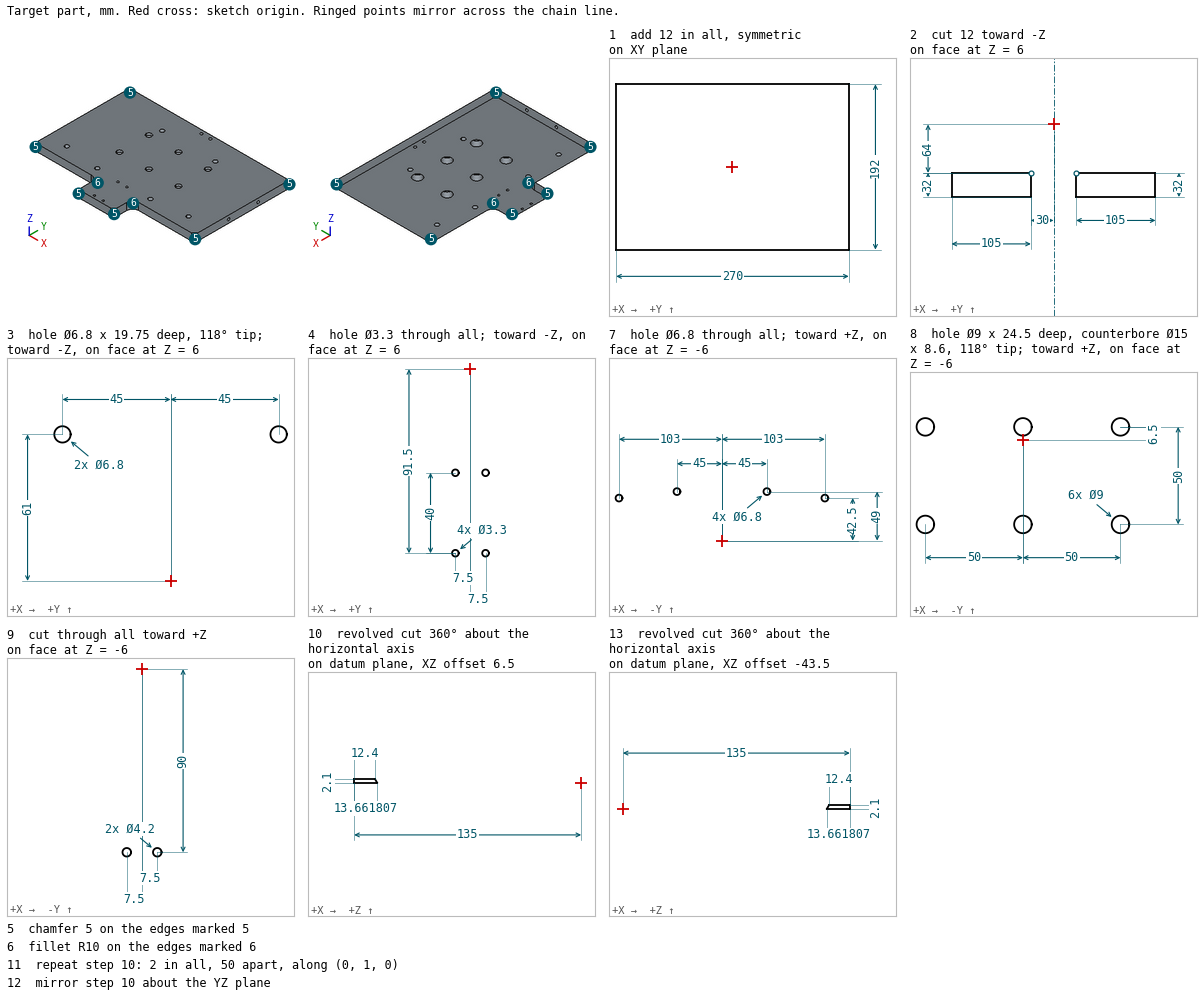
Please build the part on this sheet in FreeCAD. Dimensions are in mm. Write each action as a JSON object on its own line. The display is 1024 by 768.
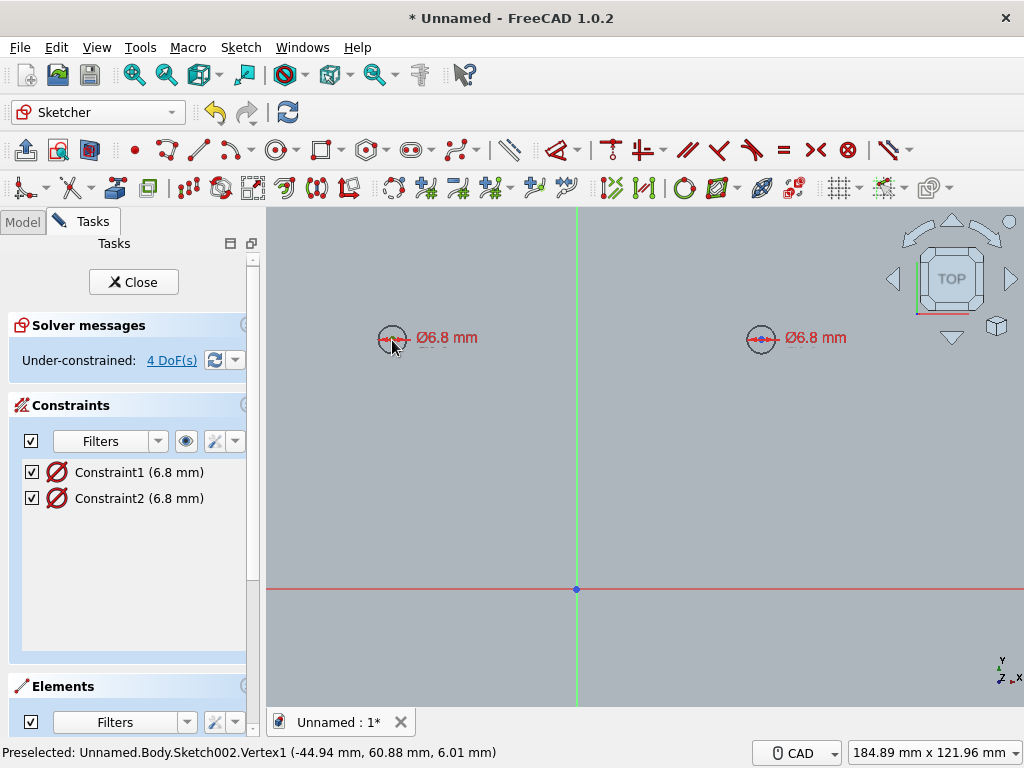
{"action": "left_click", "coordinate": [761, 340]}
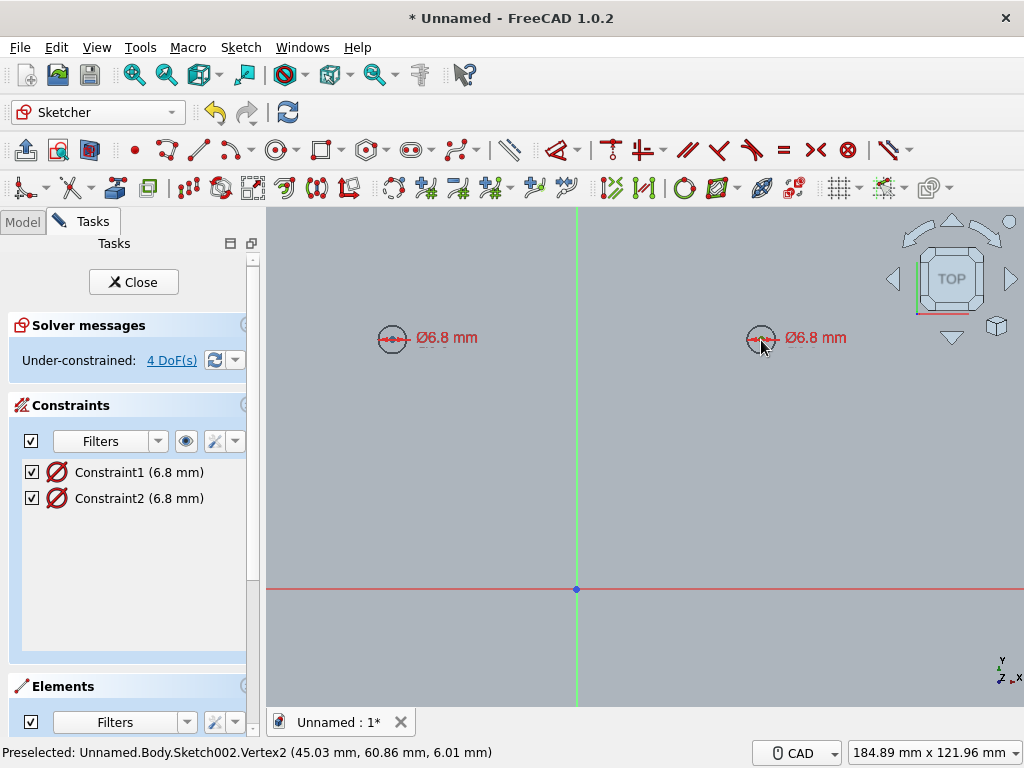
{"action": "left_click", "coordinate": [666, 150]}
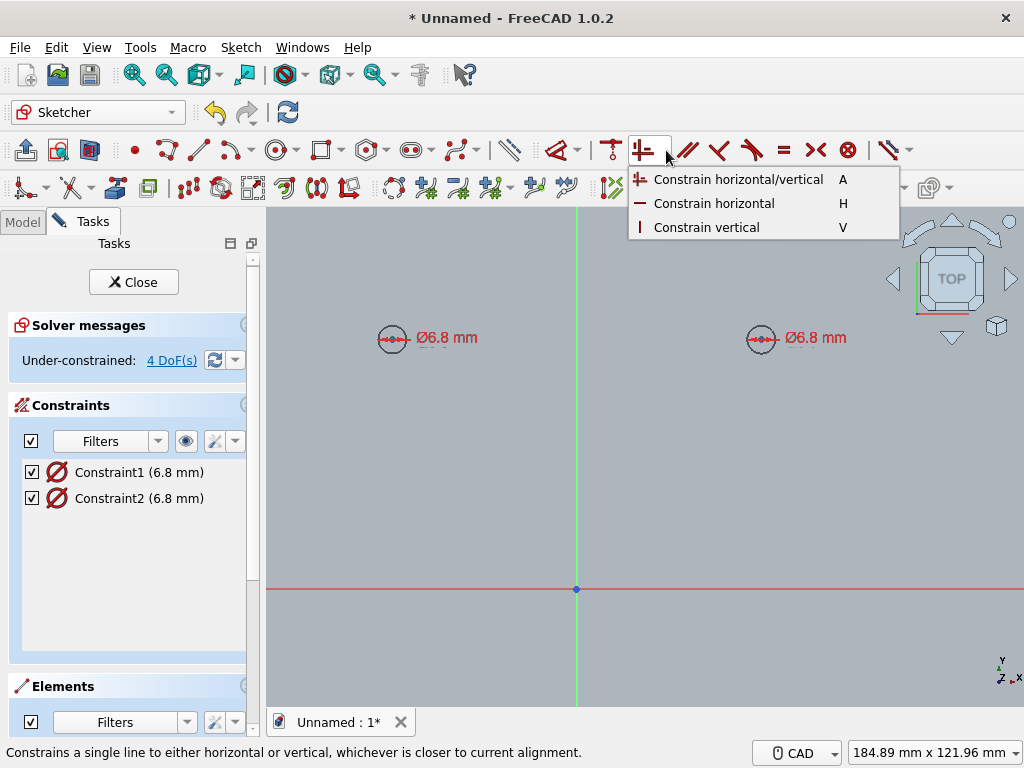
{"action": "left_click", "coordinate": [764, 203]}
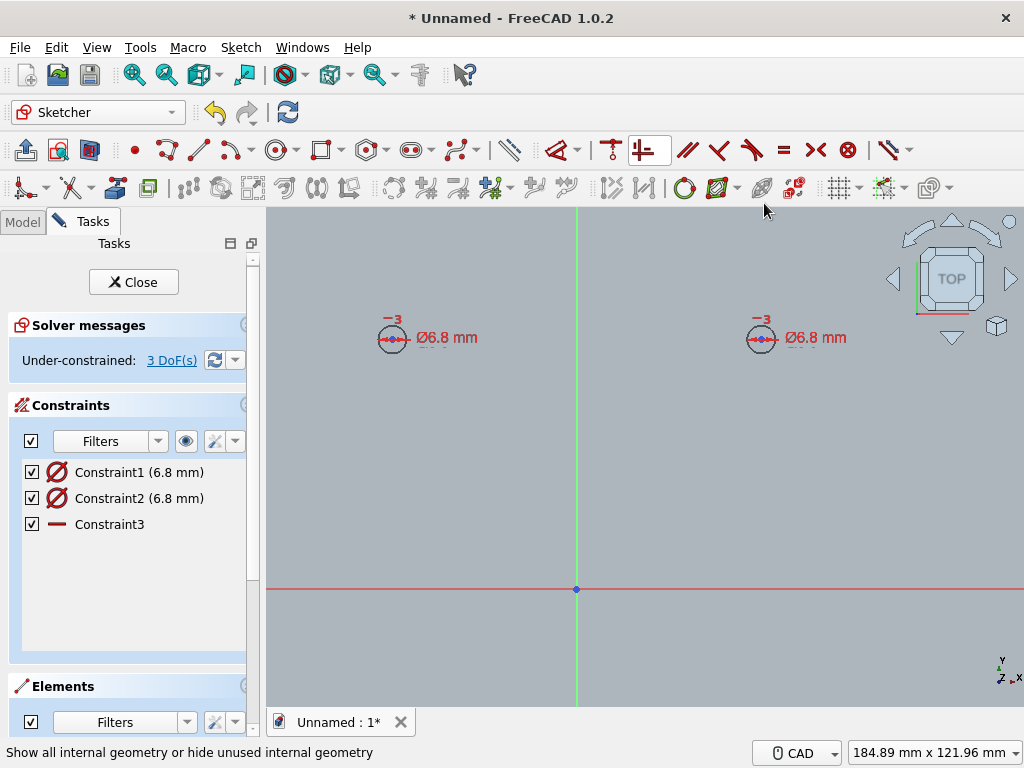
{"action": "key", "text": "d"}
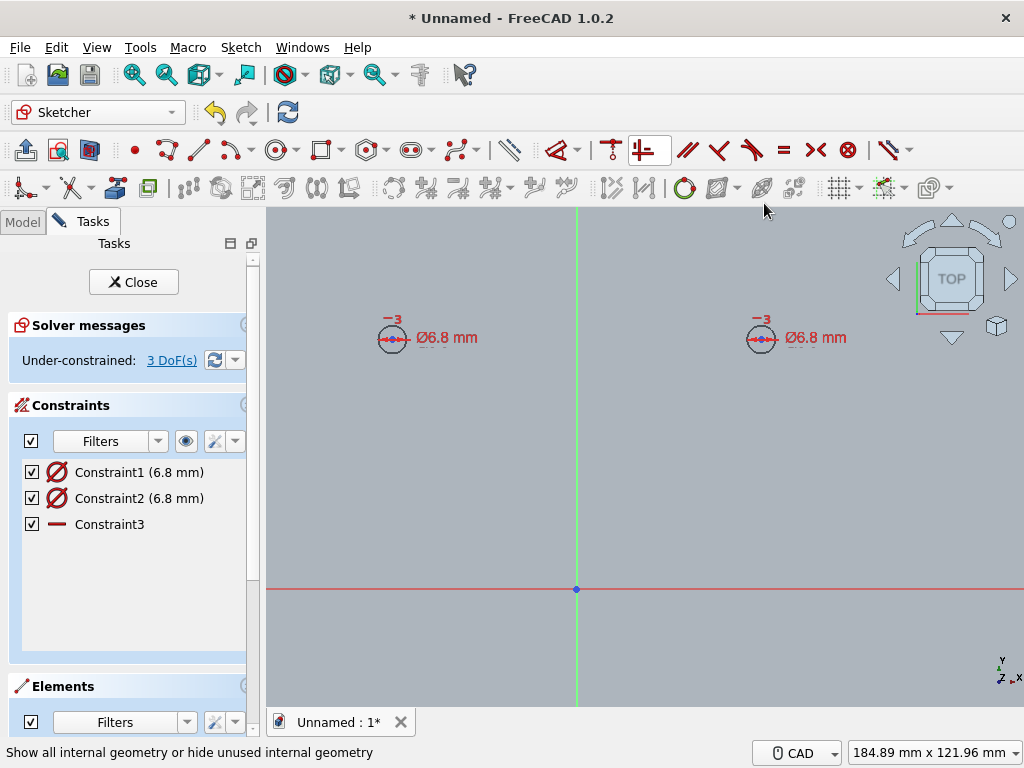
{"action": "left_click", "coordinate": [392, 340]}
{"action": "left_click", "coordinate": [485, 623]}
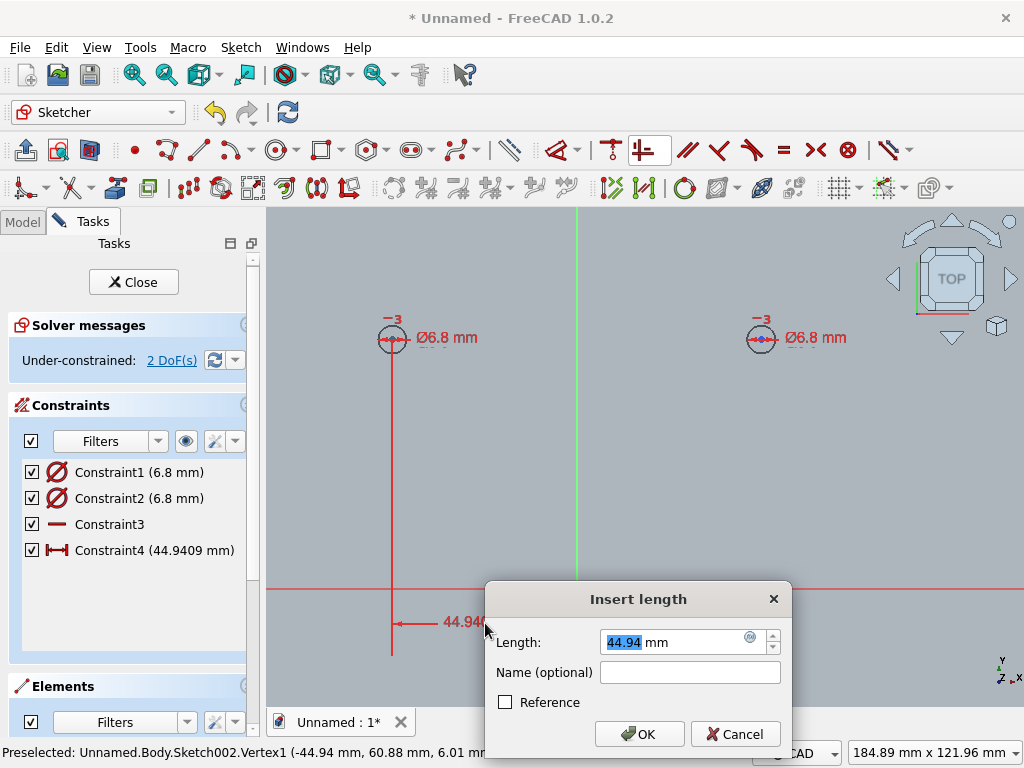
{"action": "type", "text": "45"}
{"action": "key", "text": "Return"}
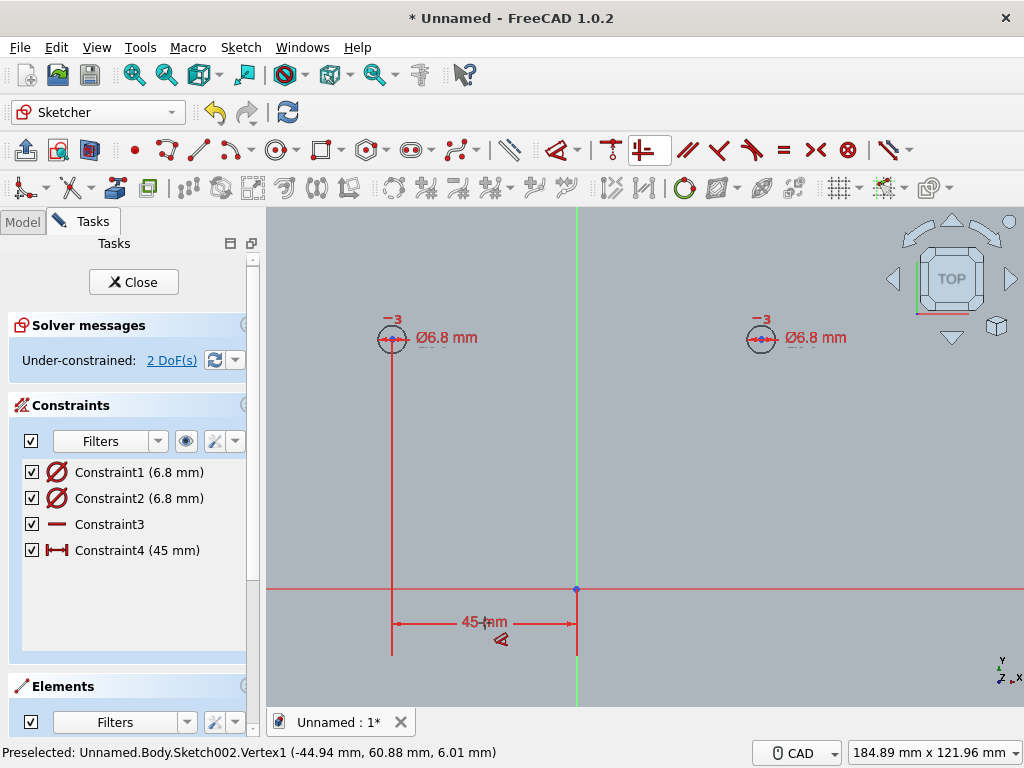
{"action": "left_click", "coordinate": [392, 340]}
{"action": "left_click", "coordinate": [358, 464]}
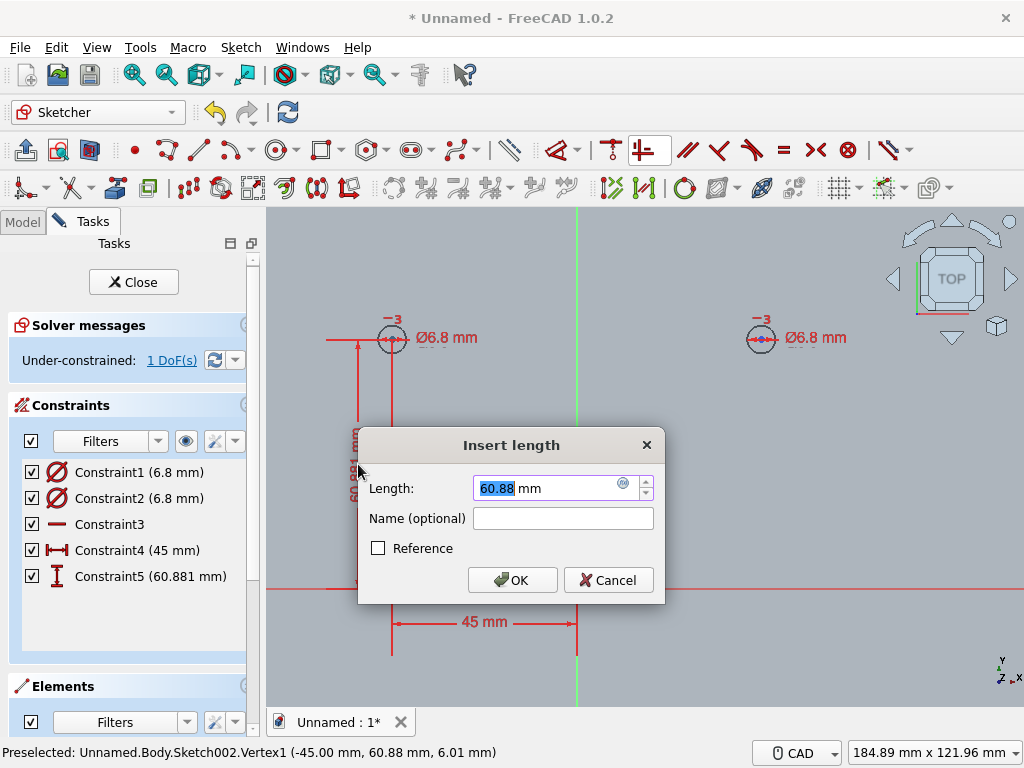
{"action": "type", "text": "61"}
{"action": "key", "text": "Return"}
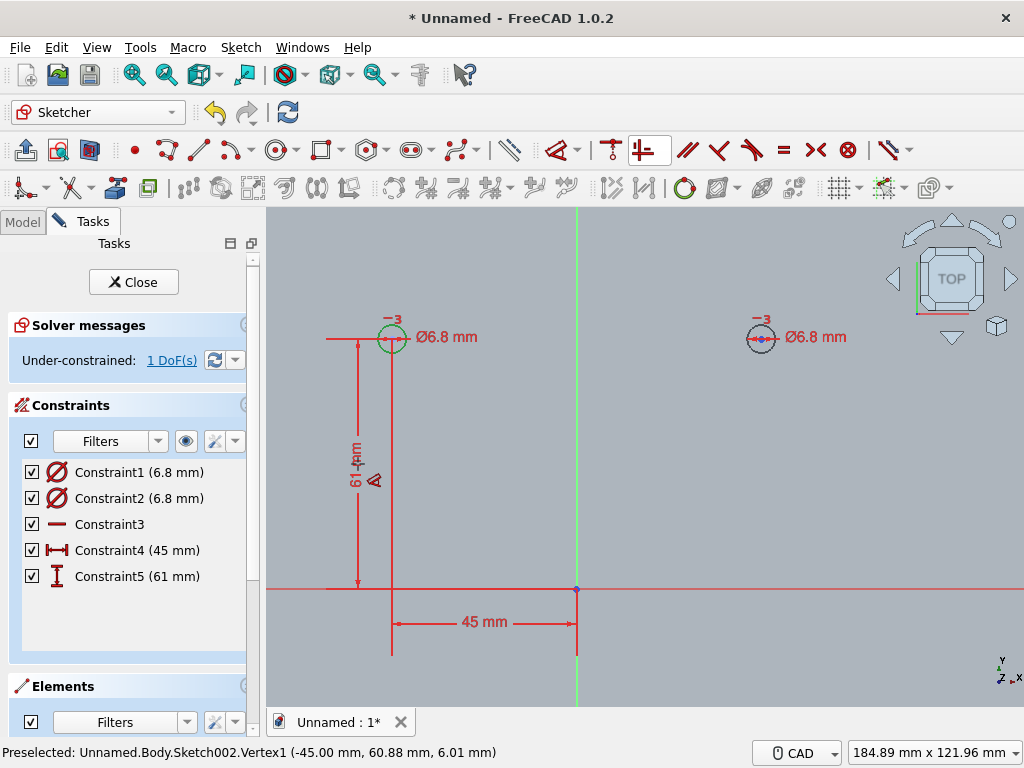
{"action": "left_click", "coordinate": [761, 339]}
{"action": "left_click", "coordinate": [669, 623]}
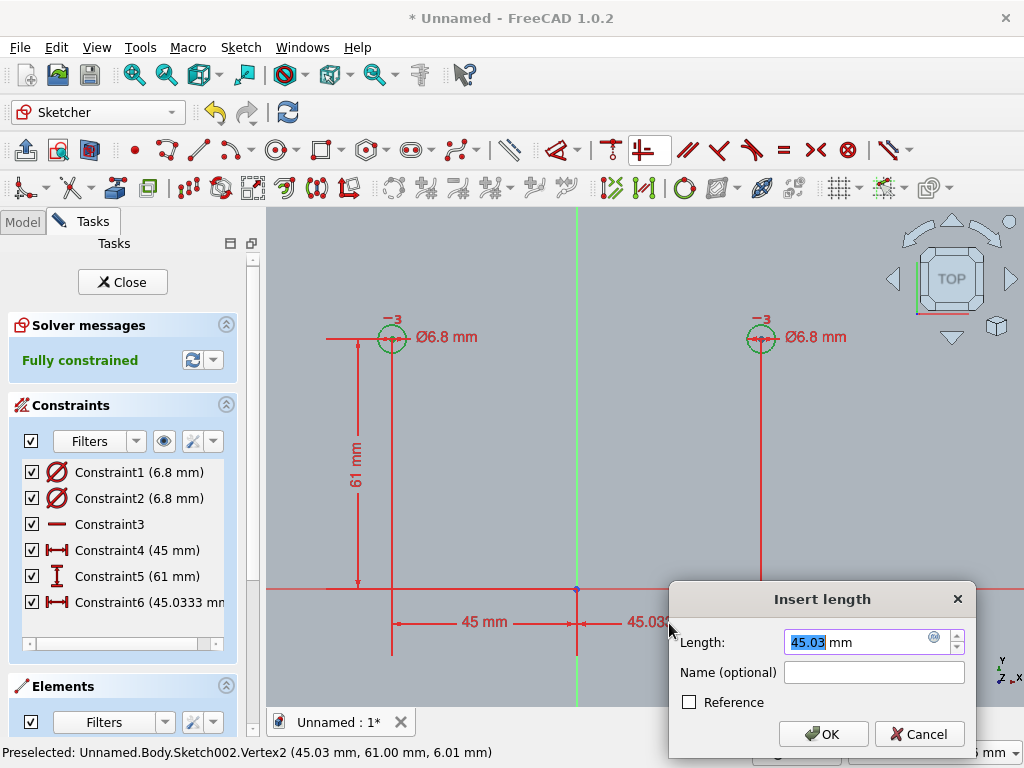
{"action": "type", "text": "45"}
{"action": "key", "text": "Return"}
{"action": "key", "text": "Escape"}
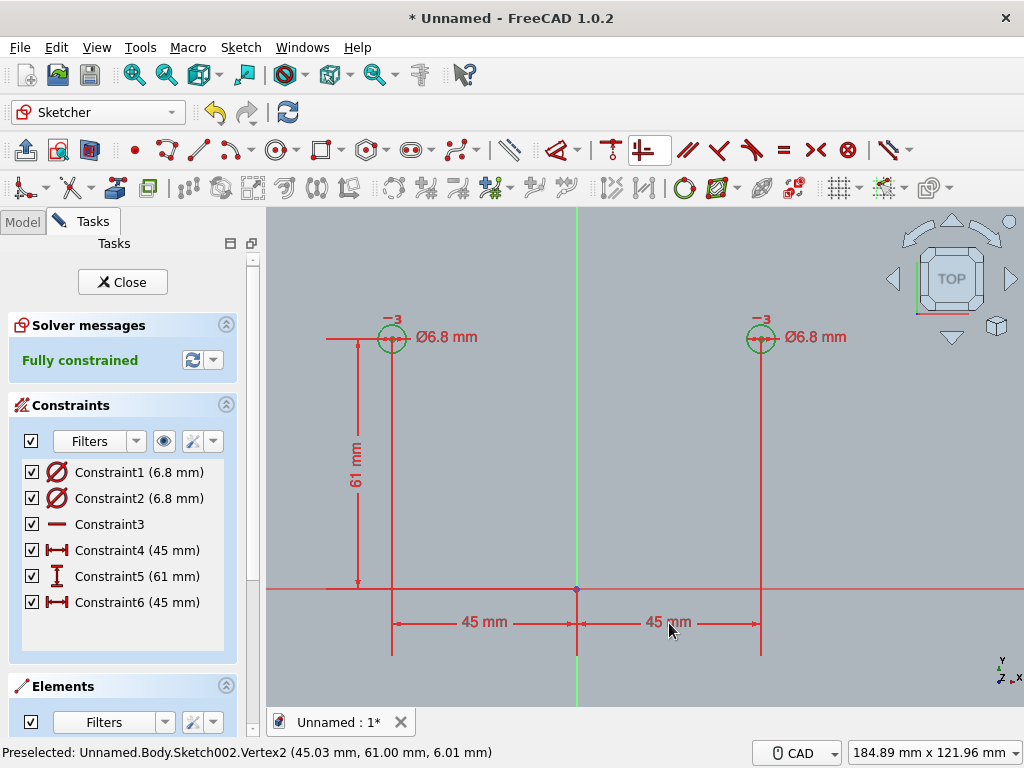
{"action": "left_click", "coordinate": [123, 282]}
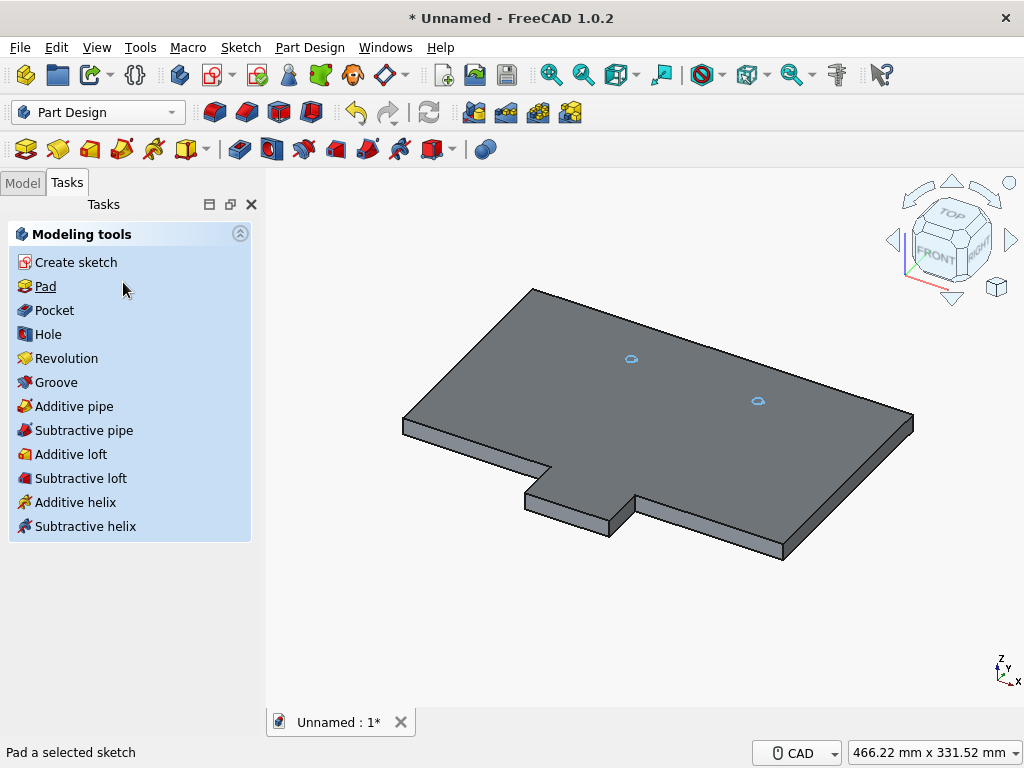
{"action": "left_click", "coordinate": [272, 150]}